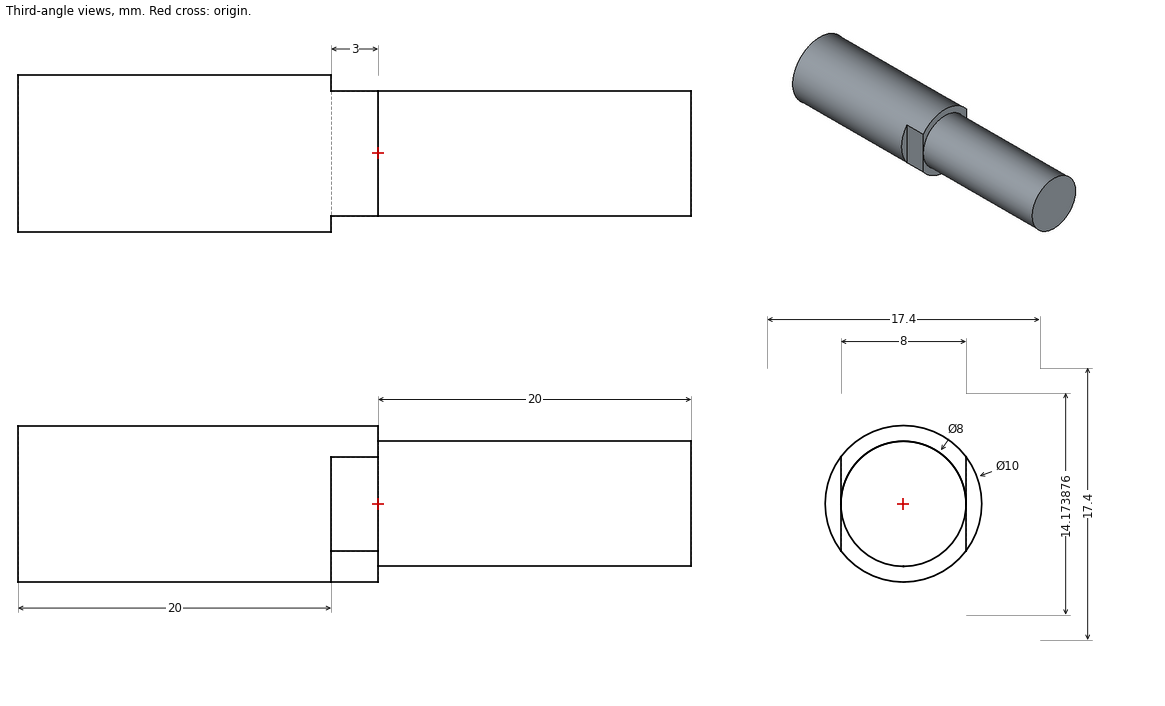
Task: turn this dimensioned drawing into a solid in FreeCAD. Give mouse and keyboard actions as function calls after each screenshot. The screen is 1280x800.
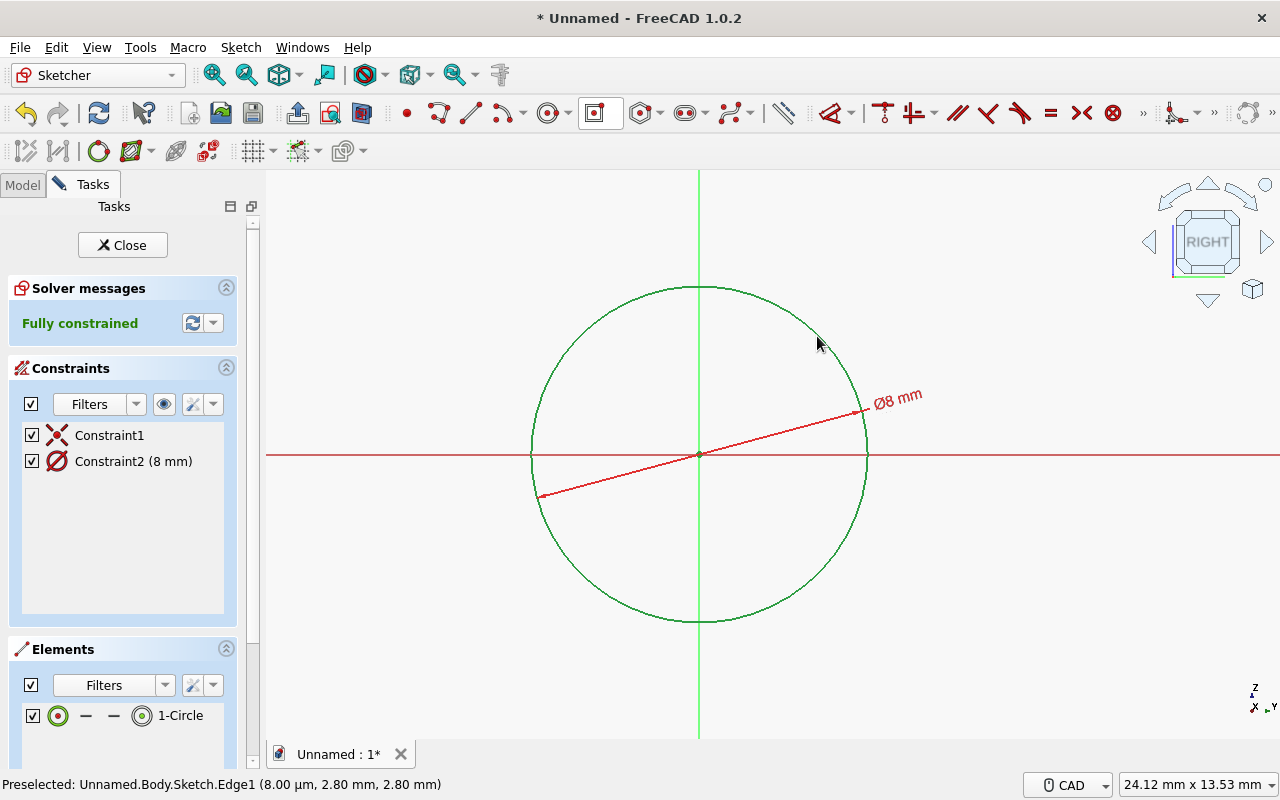
click(123, 245)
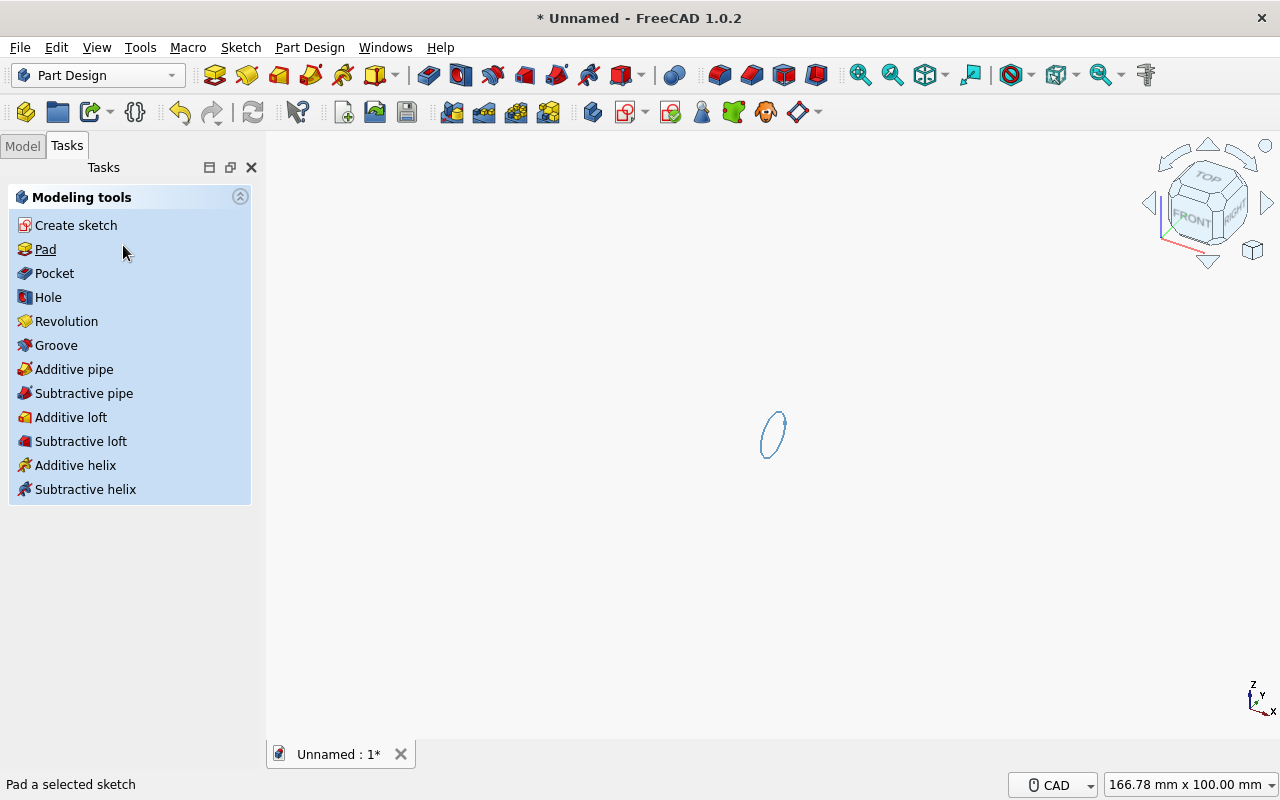
click(216, 76)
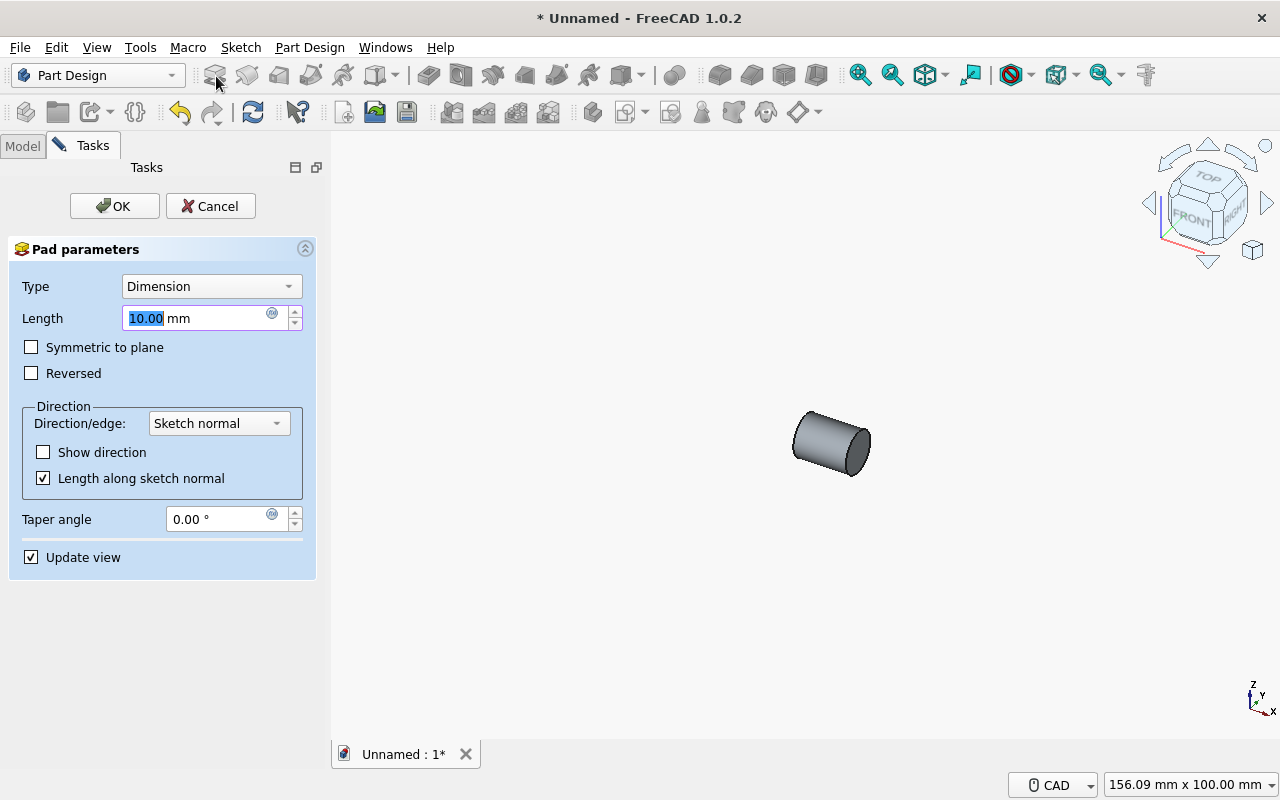
text(20)
key(Tab)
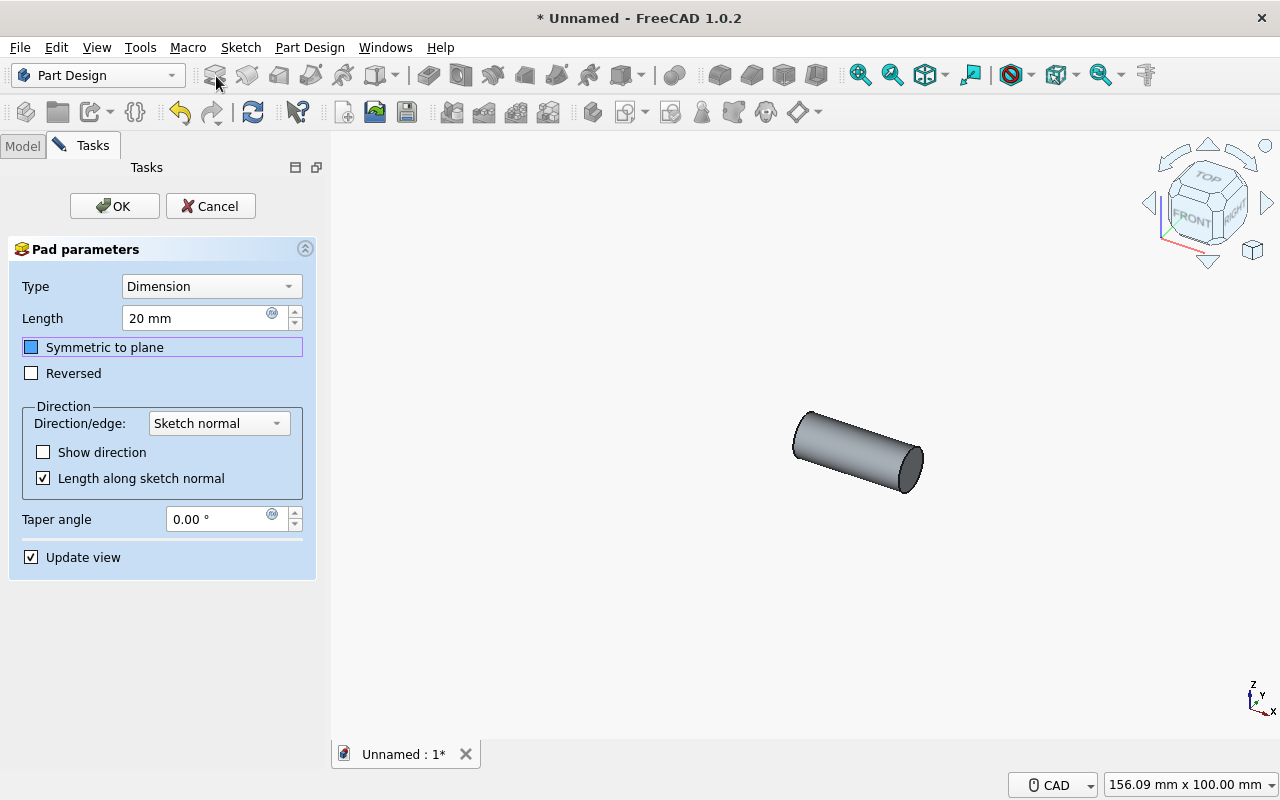
click(115, 206)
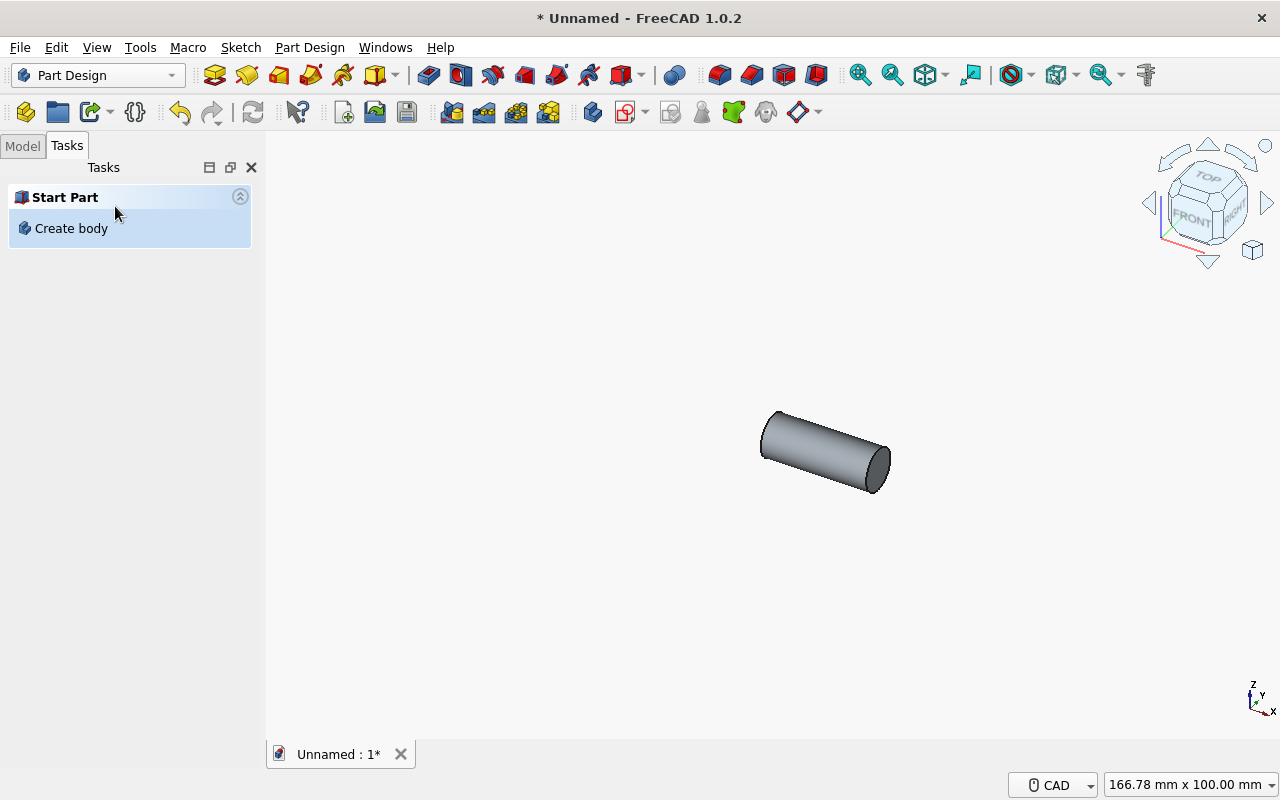
key(v)
key(f)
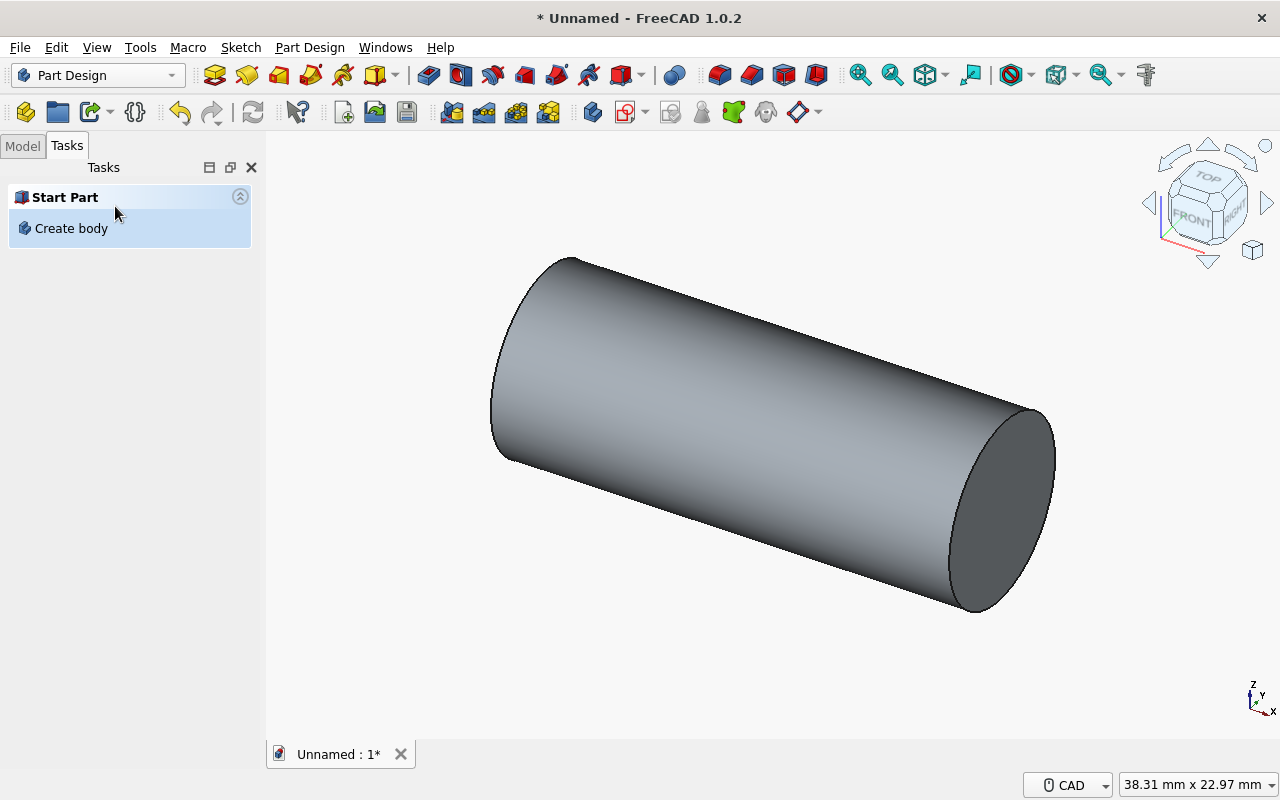
key(6)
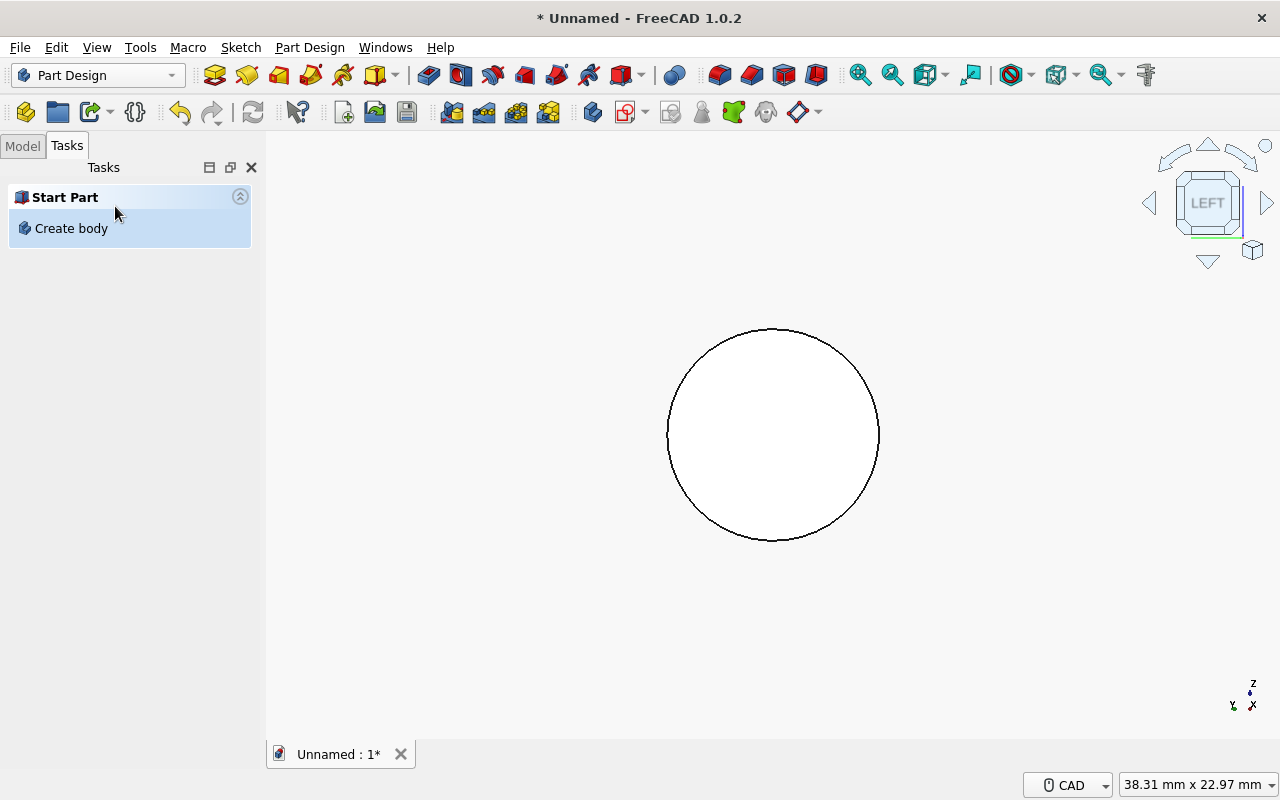
key(v)
key(f)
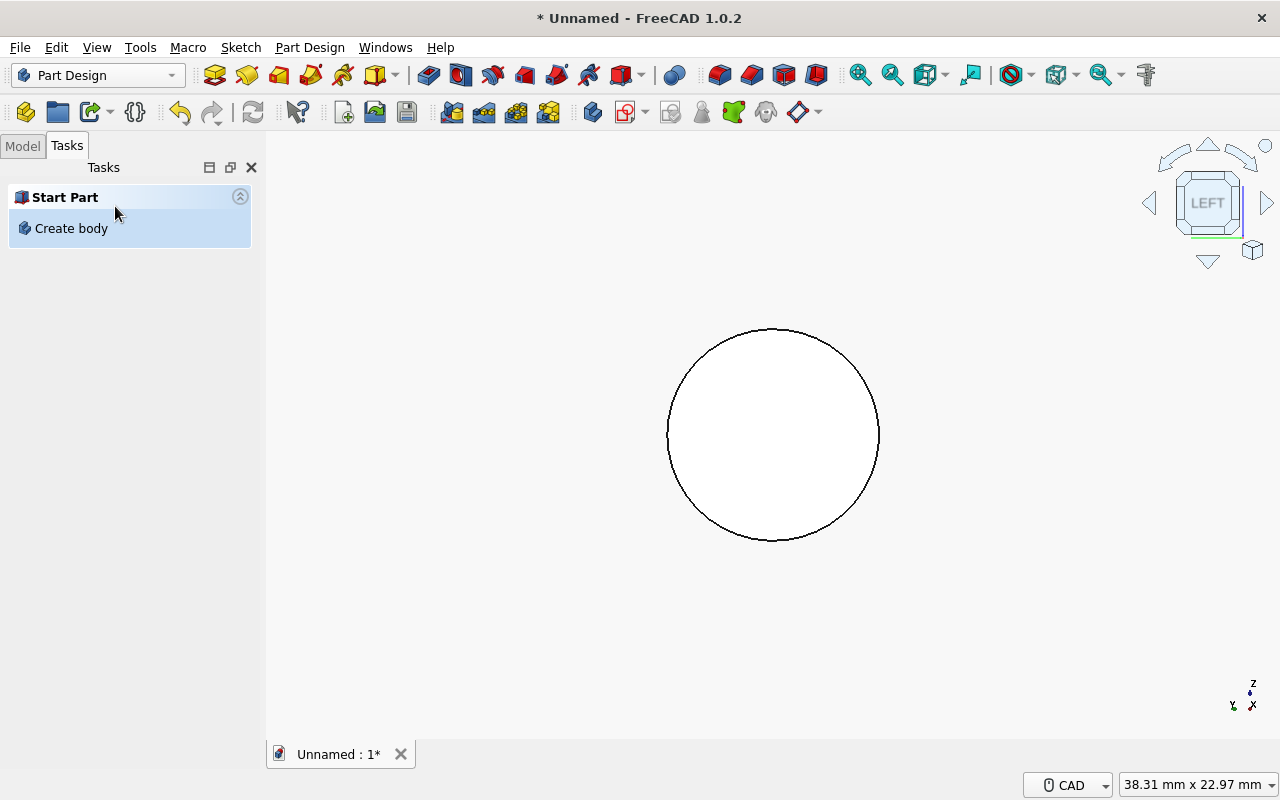
click(773, 434)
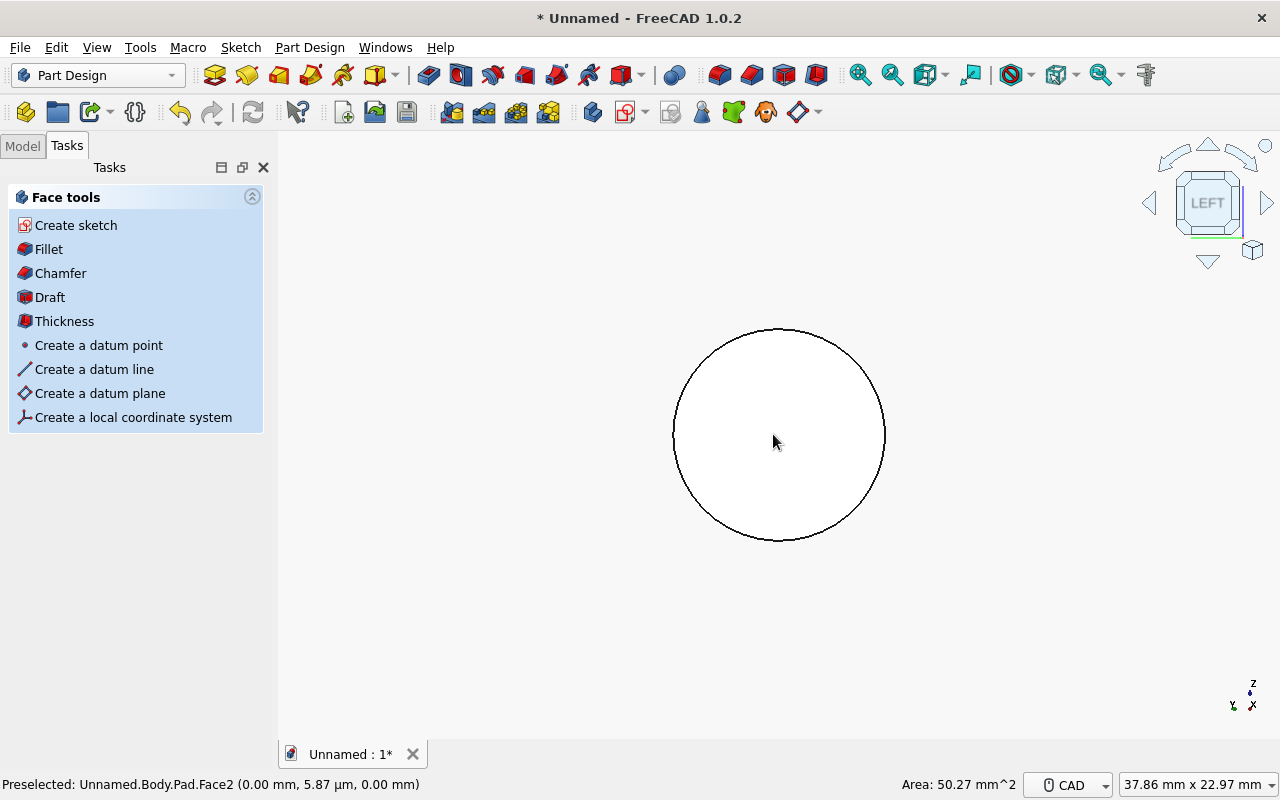
click(626, 112)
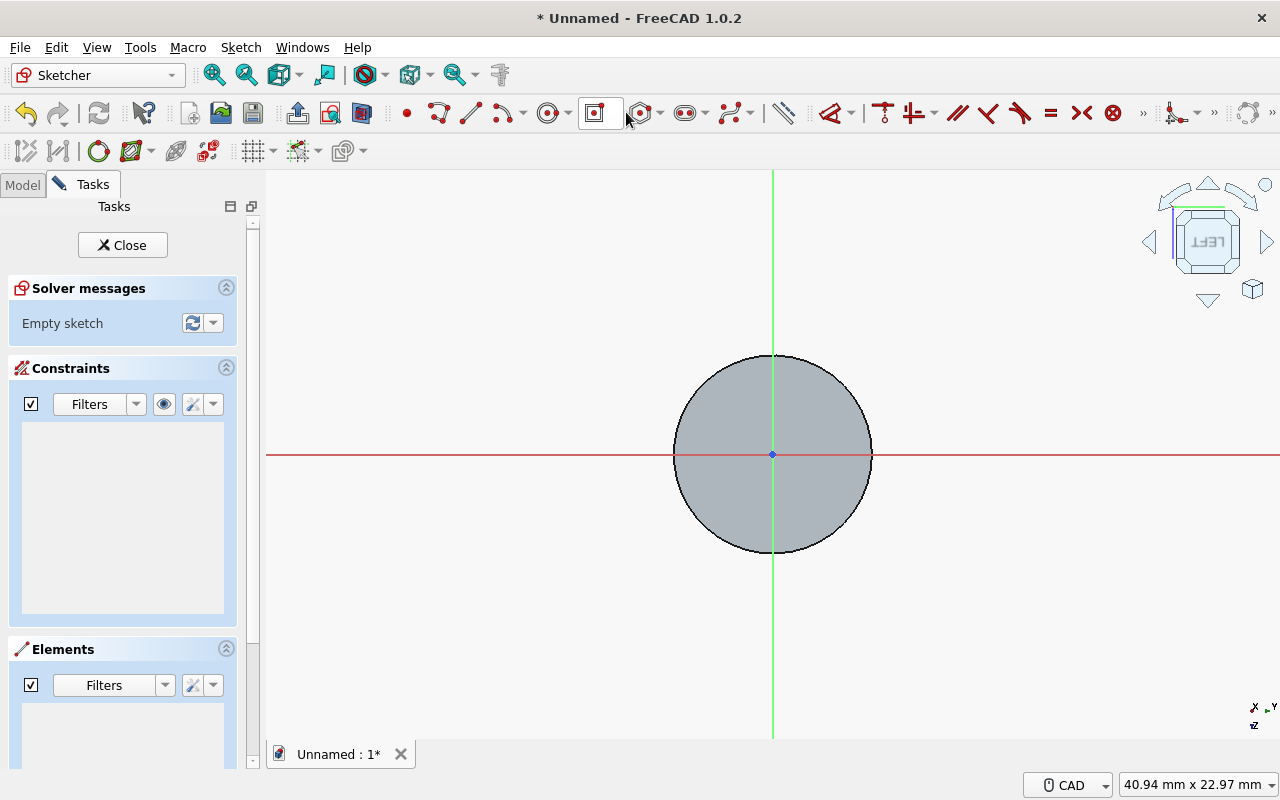
scroll(912, 455, up, 2)